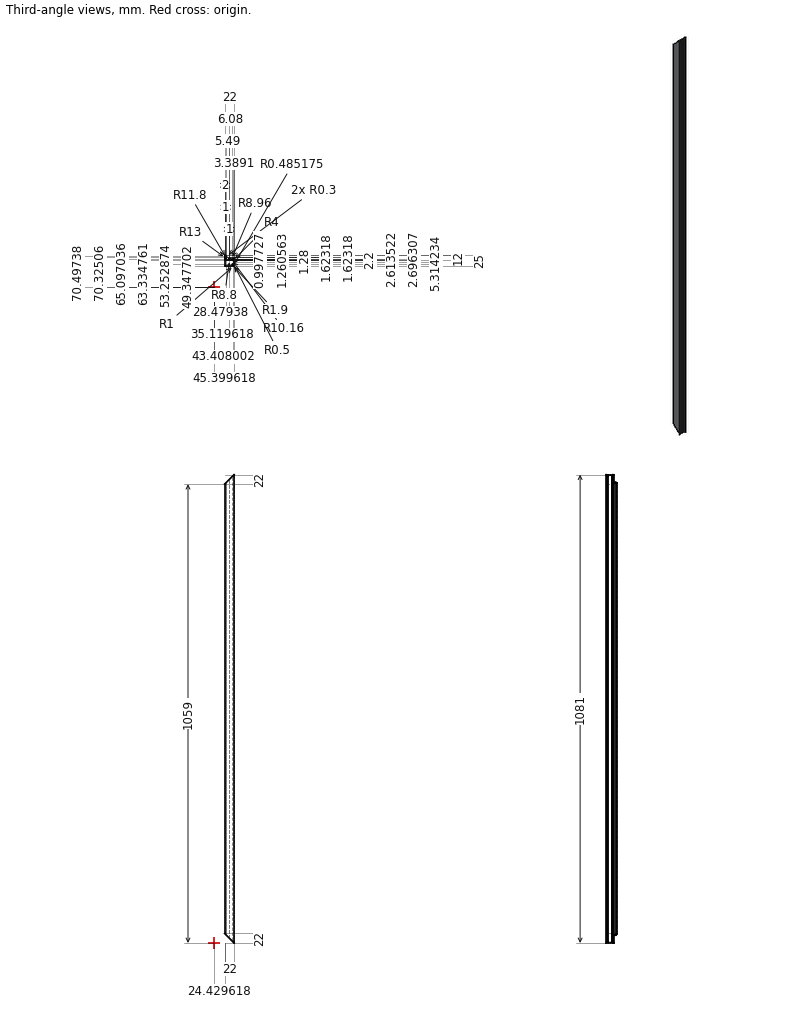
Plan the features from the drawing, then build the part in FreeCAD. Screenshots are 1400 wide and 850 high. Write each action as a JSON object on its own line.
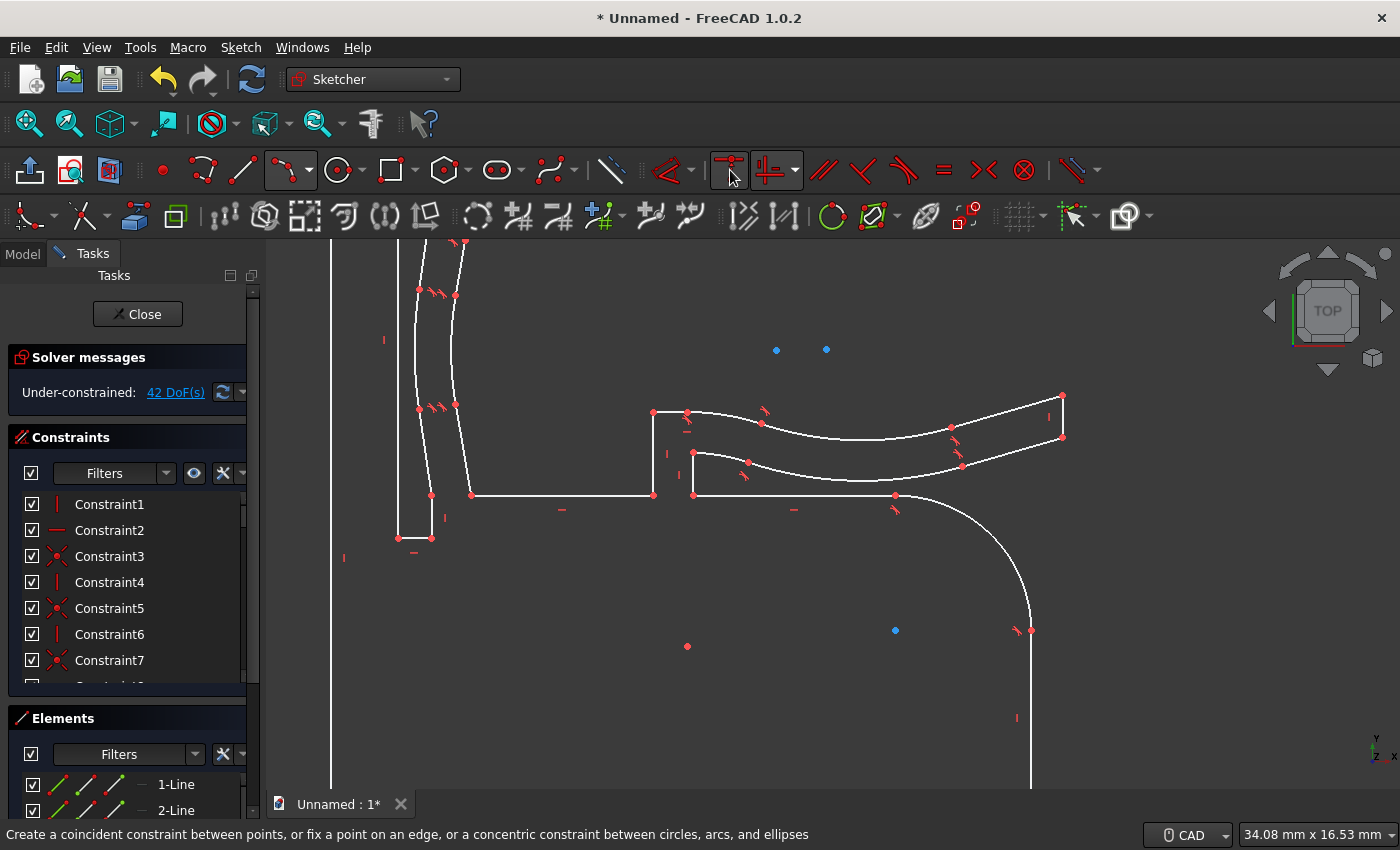
{"action": "left_click", "coordinate": [452, 328]}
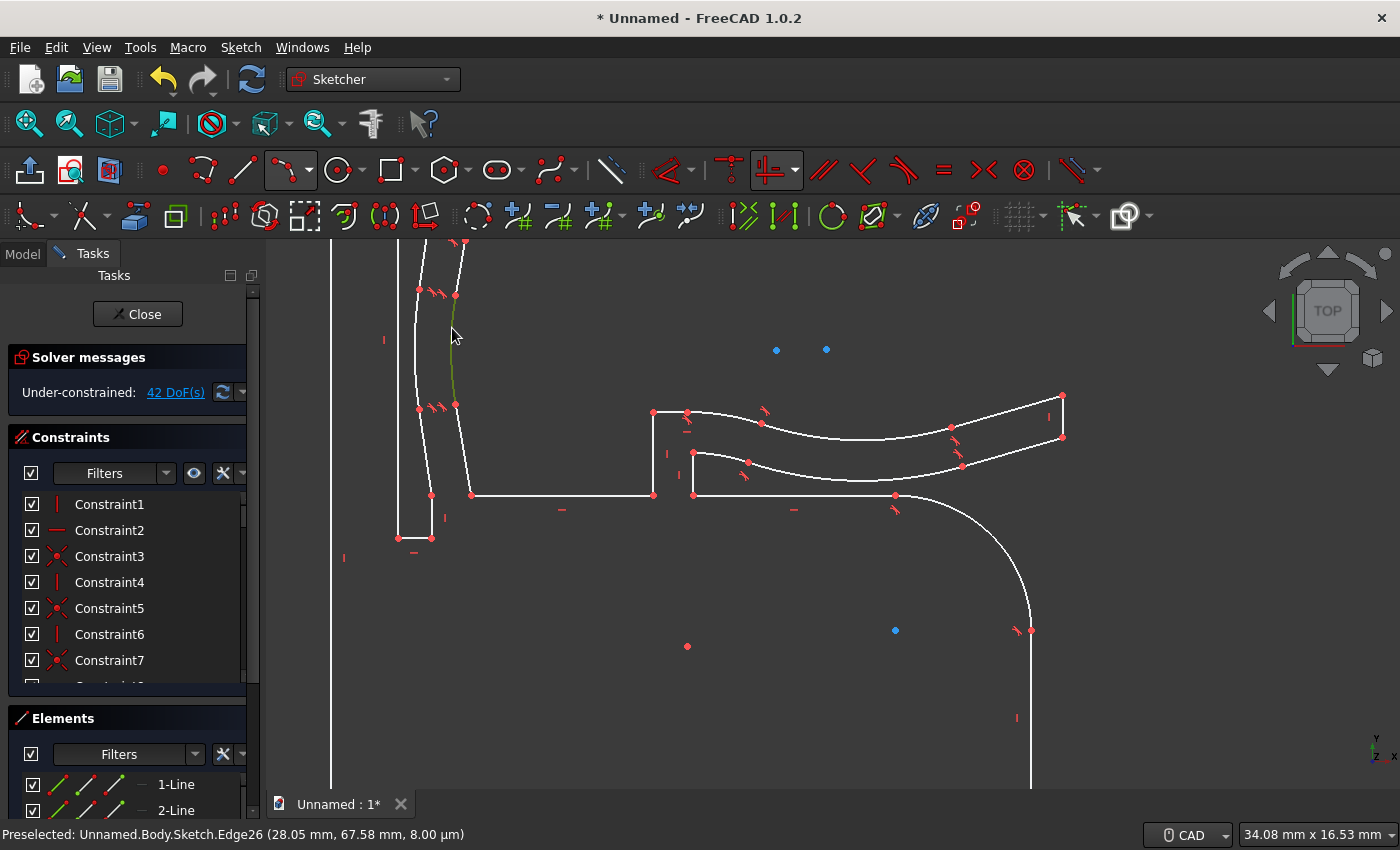
{"action": "left_click", "coordinate": [415, 325]}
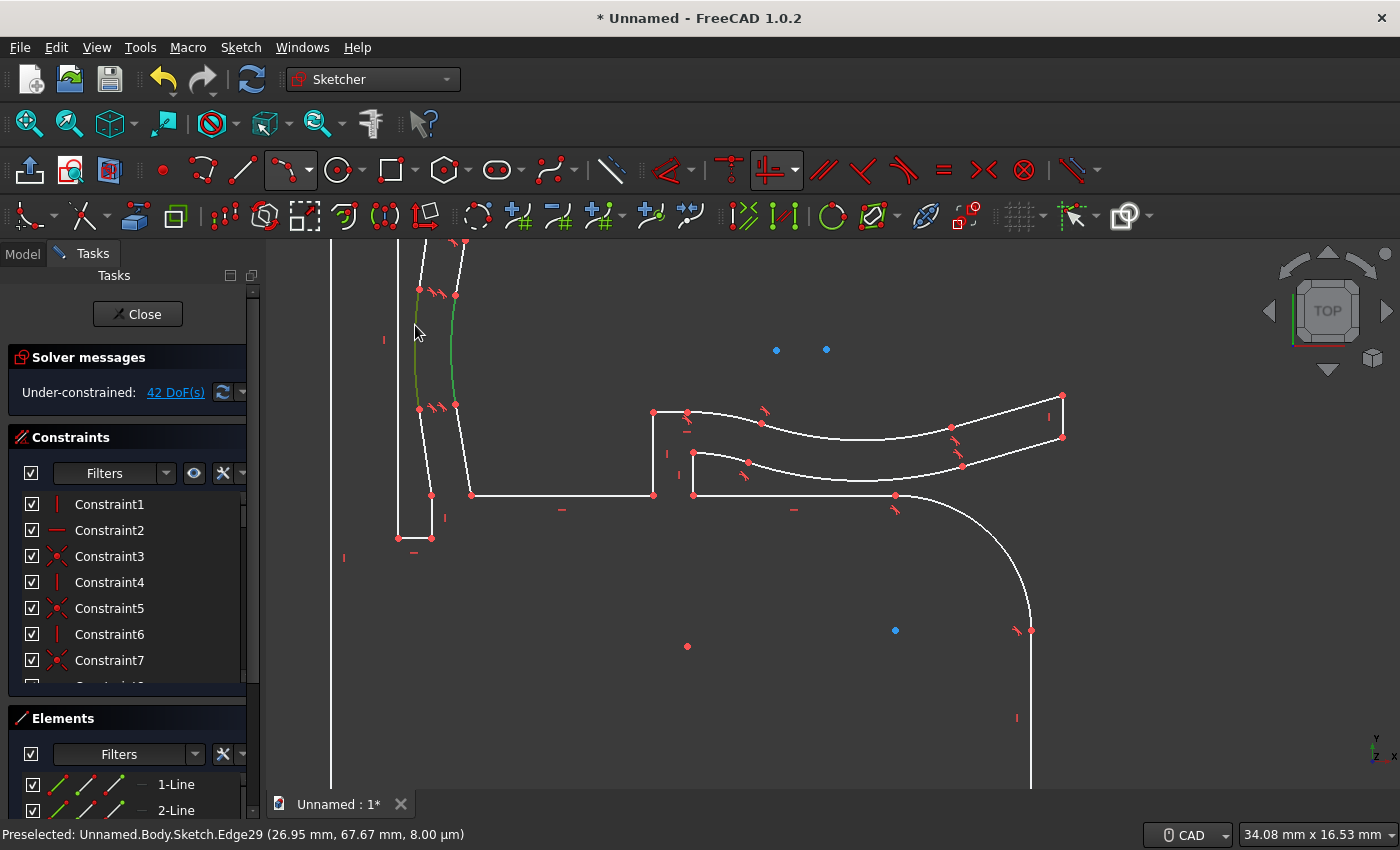
{"action": "left_click", "coordinate": [730, 170]}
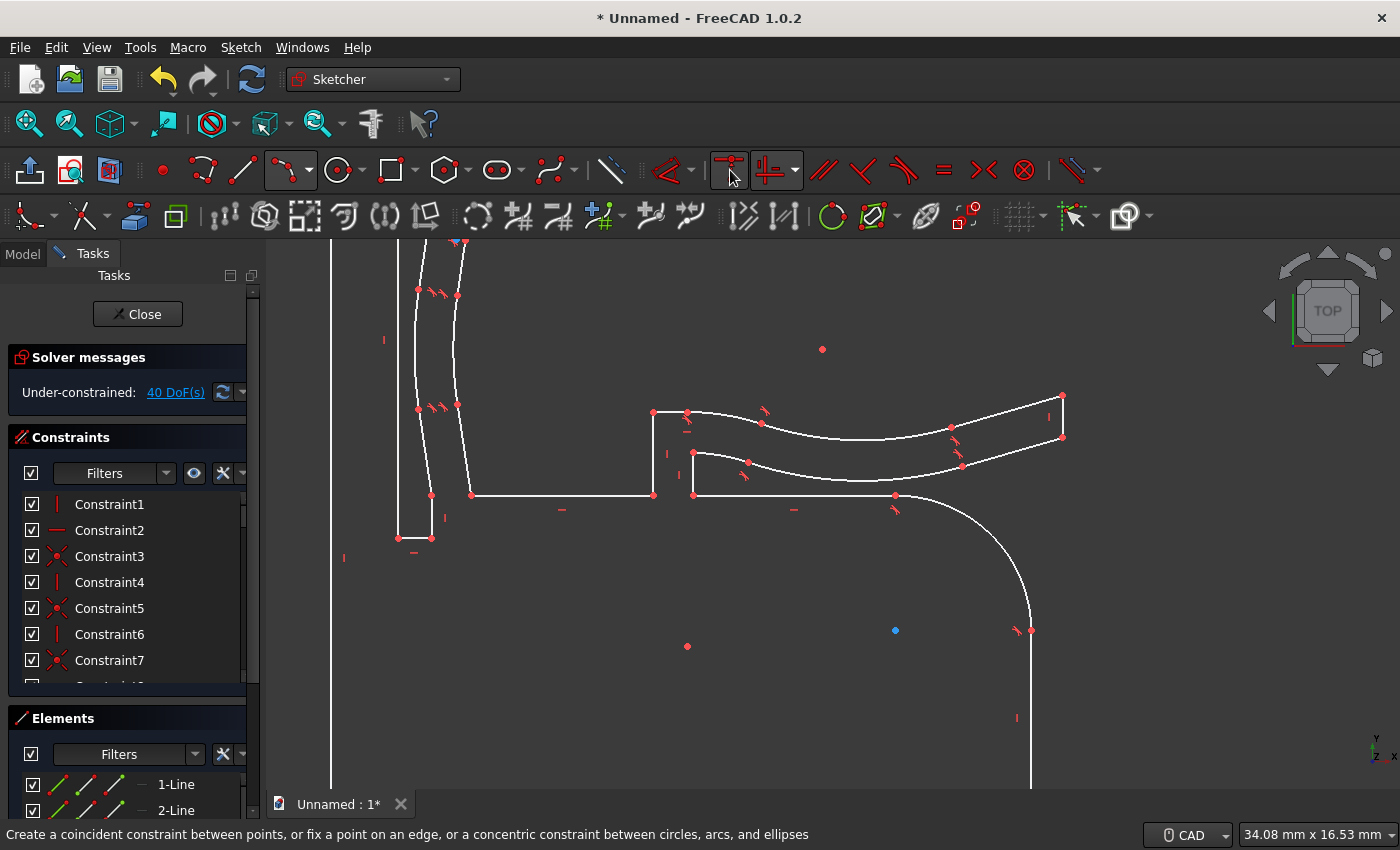
{"action": "scroll", "coordinate": [819, 481], "scroll_direction": "down", "scroll_amount": 4}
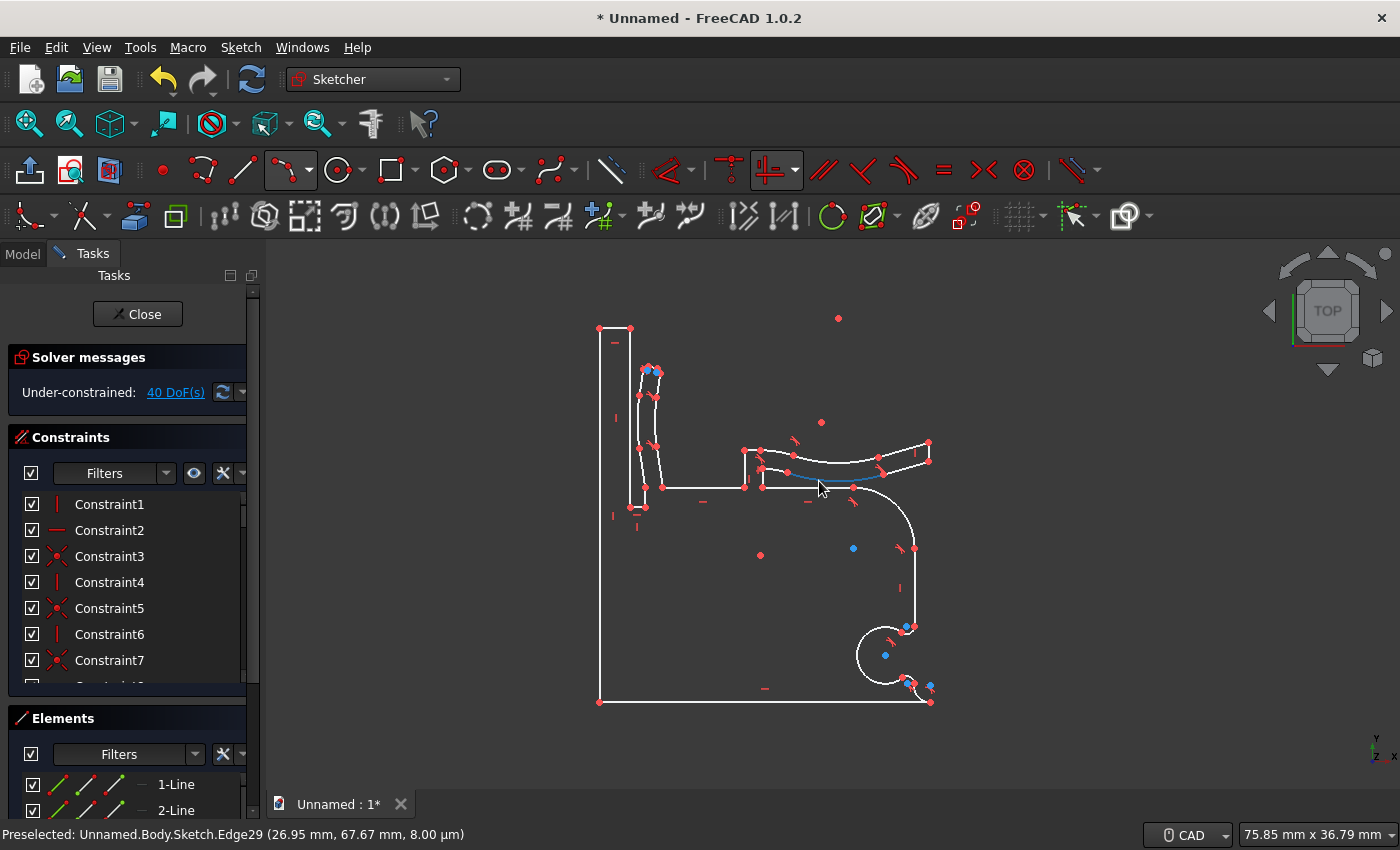
{"action": "scroll", "coordinate": [660, 370], "scroll_direction": "up", "scroll_amount": 8}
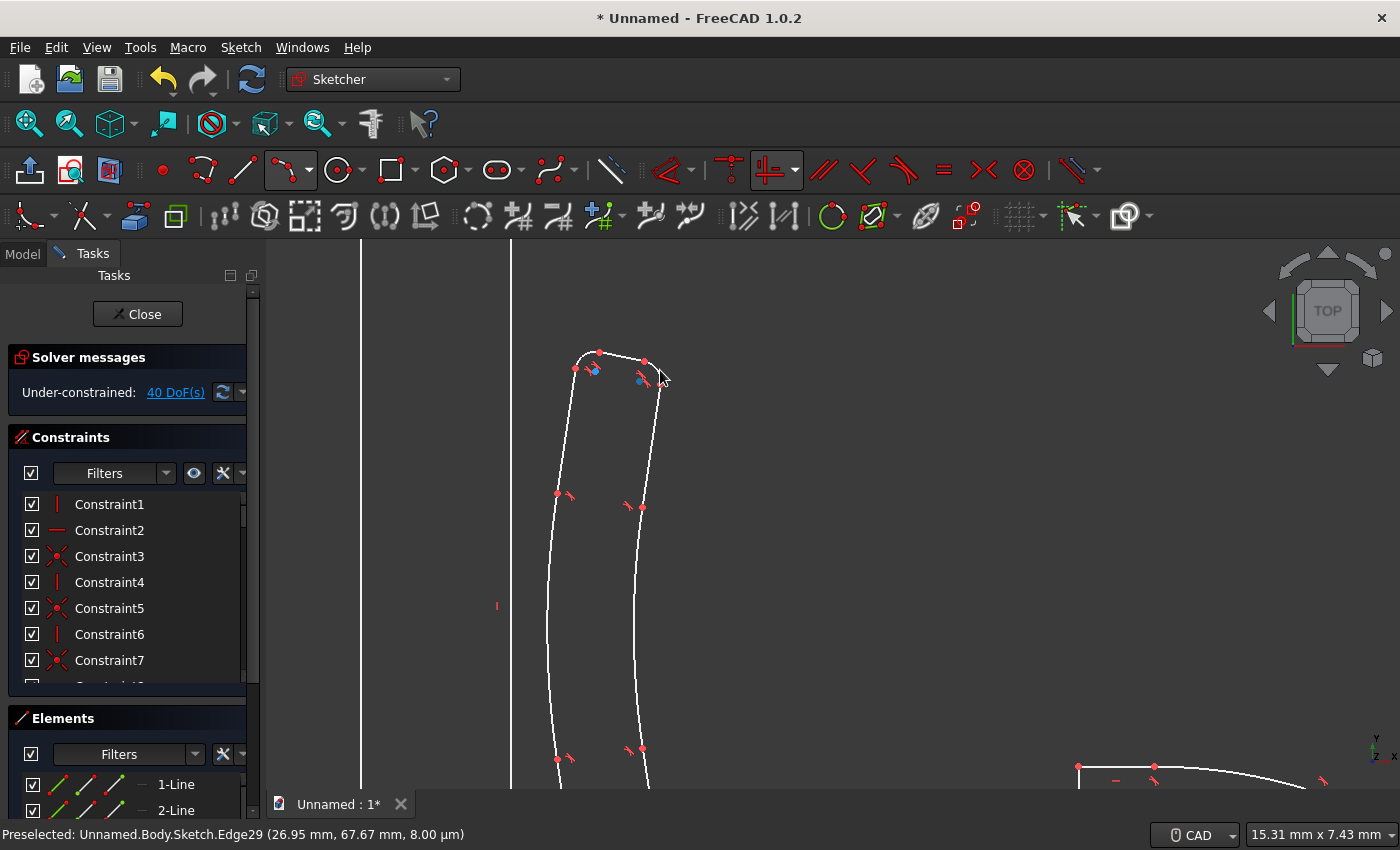
{"action": "left_click", "coordinate": [657, 370]}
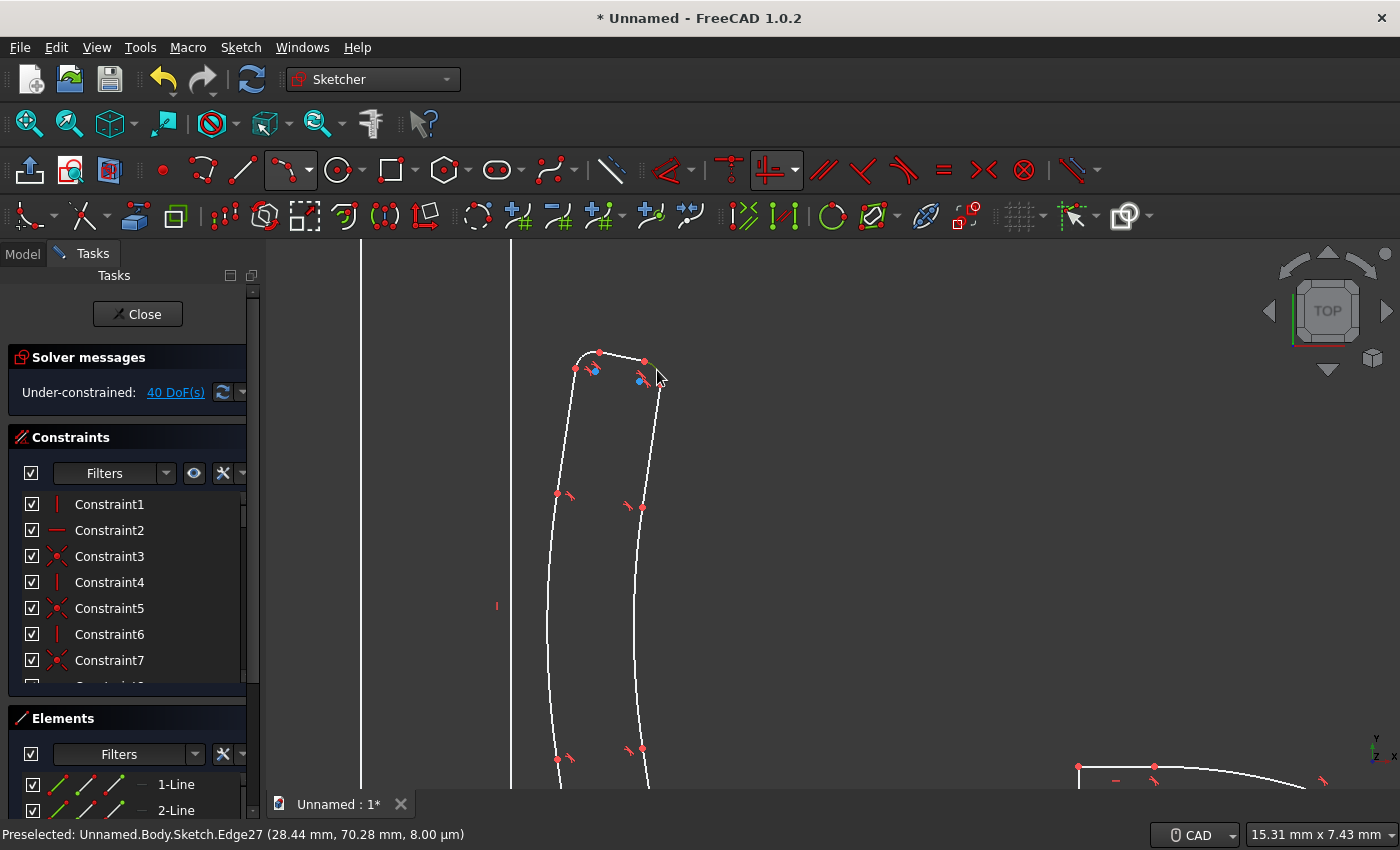
{"action": "scroll", "coordinate": [590, 352], "scroll_direction": "up", "scroll_amount": 2}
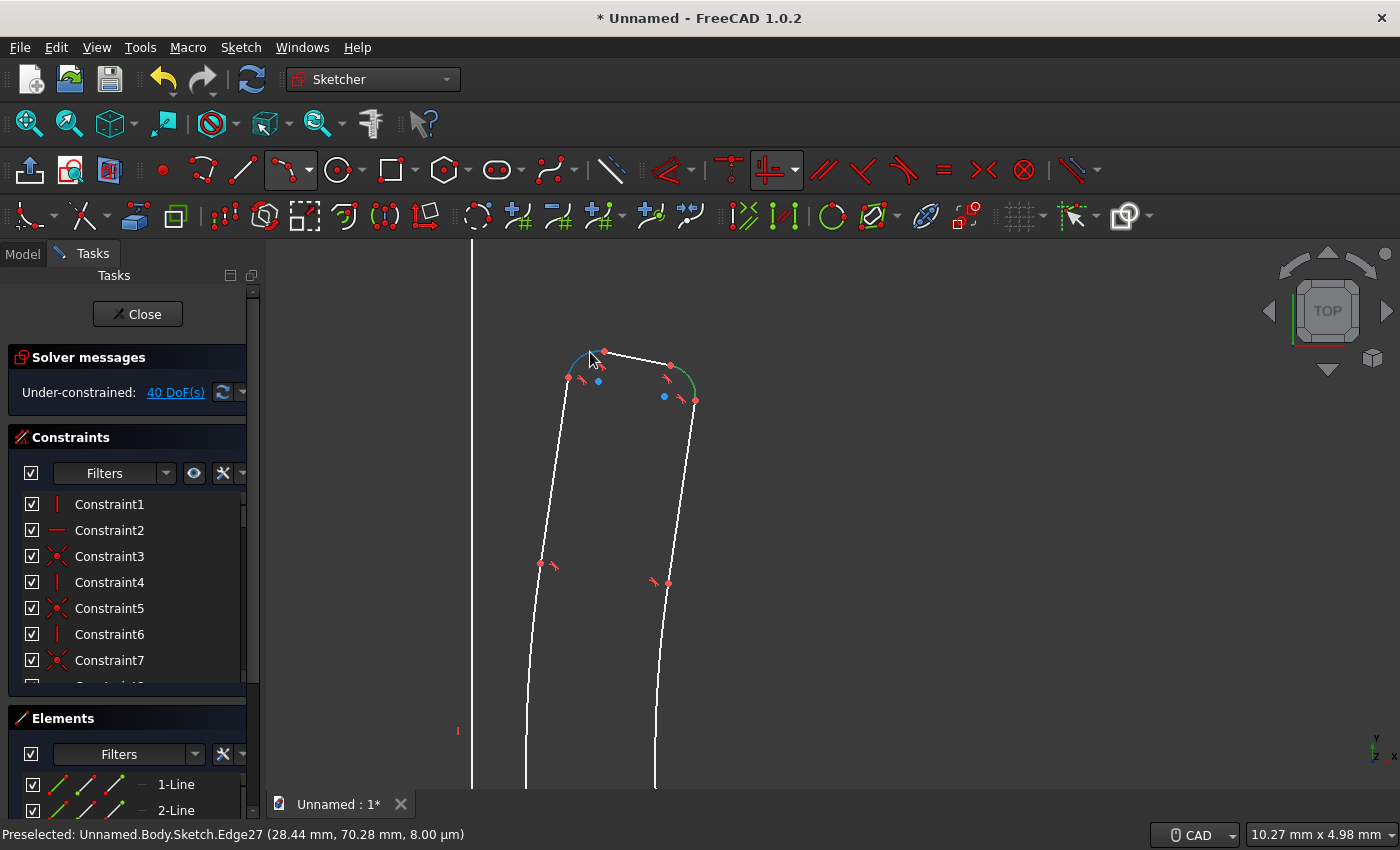
{"action": "left_click", "coordinate": [590, 353]}